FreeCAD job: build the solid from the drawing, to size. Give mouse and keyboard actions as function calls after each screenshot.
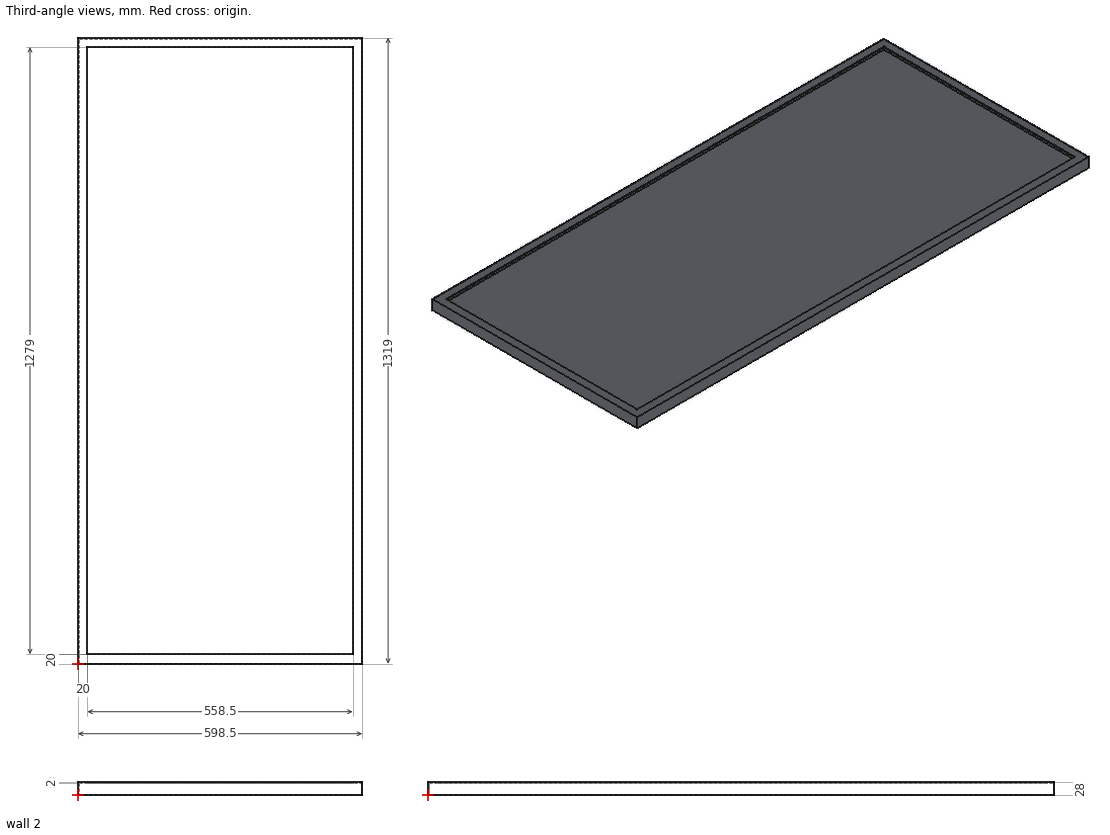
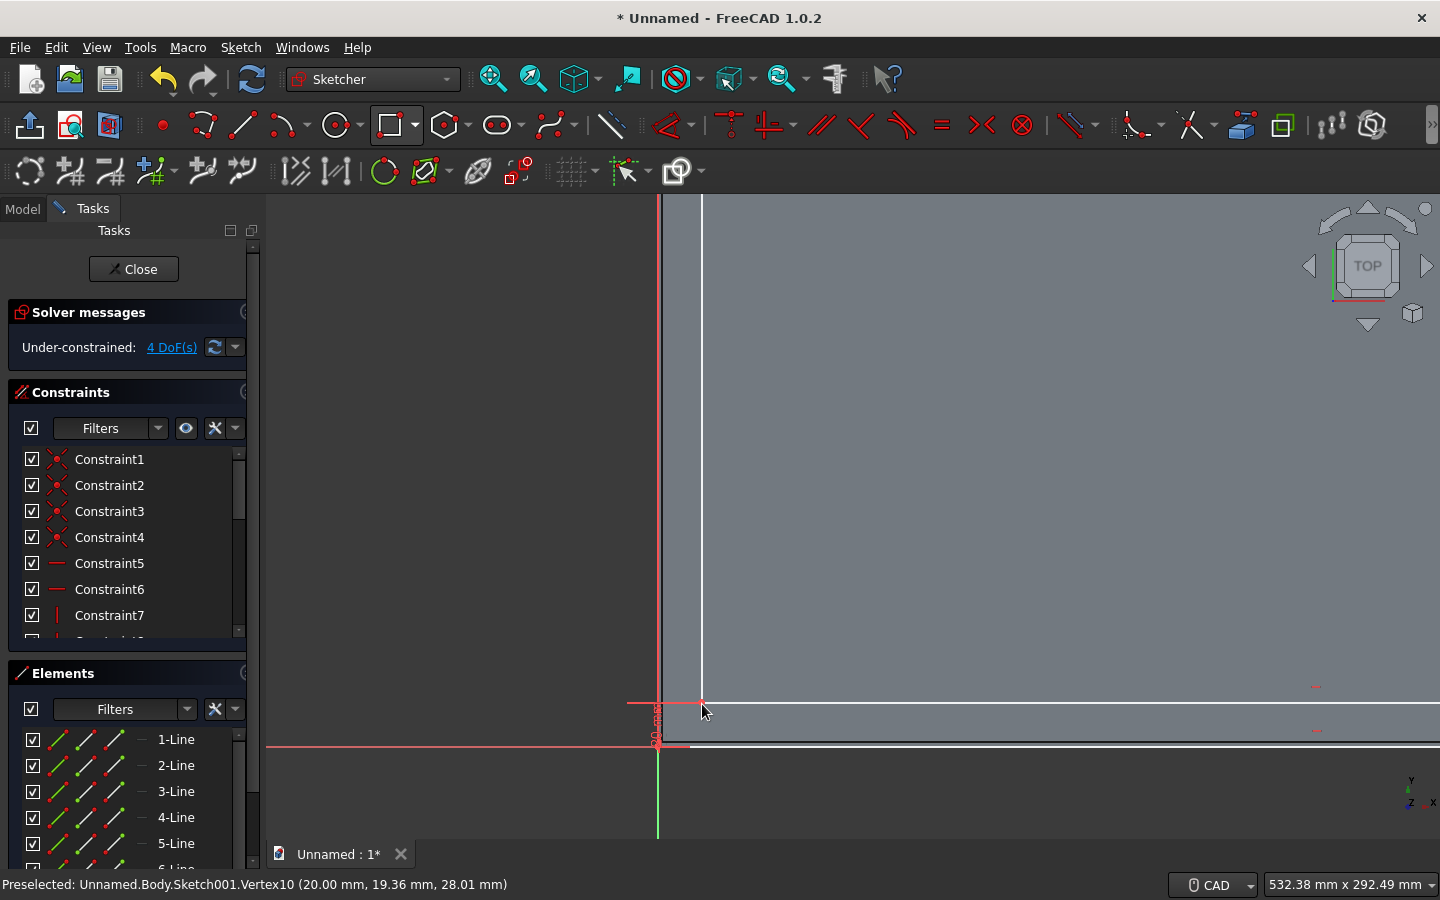
scroll(701, 708, down, 10)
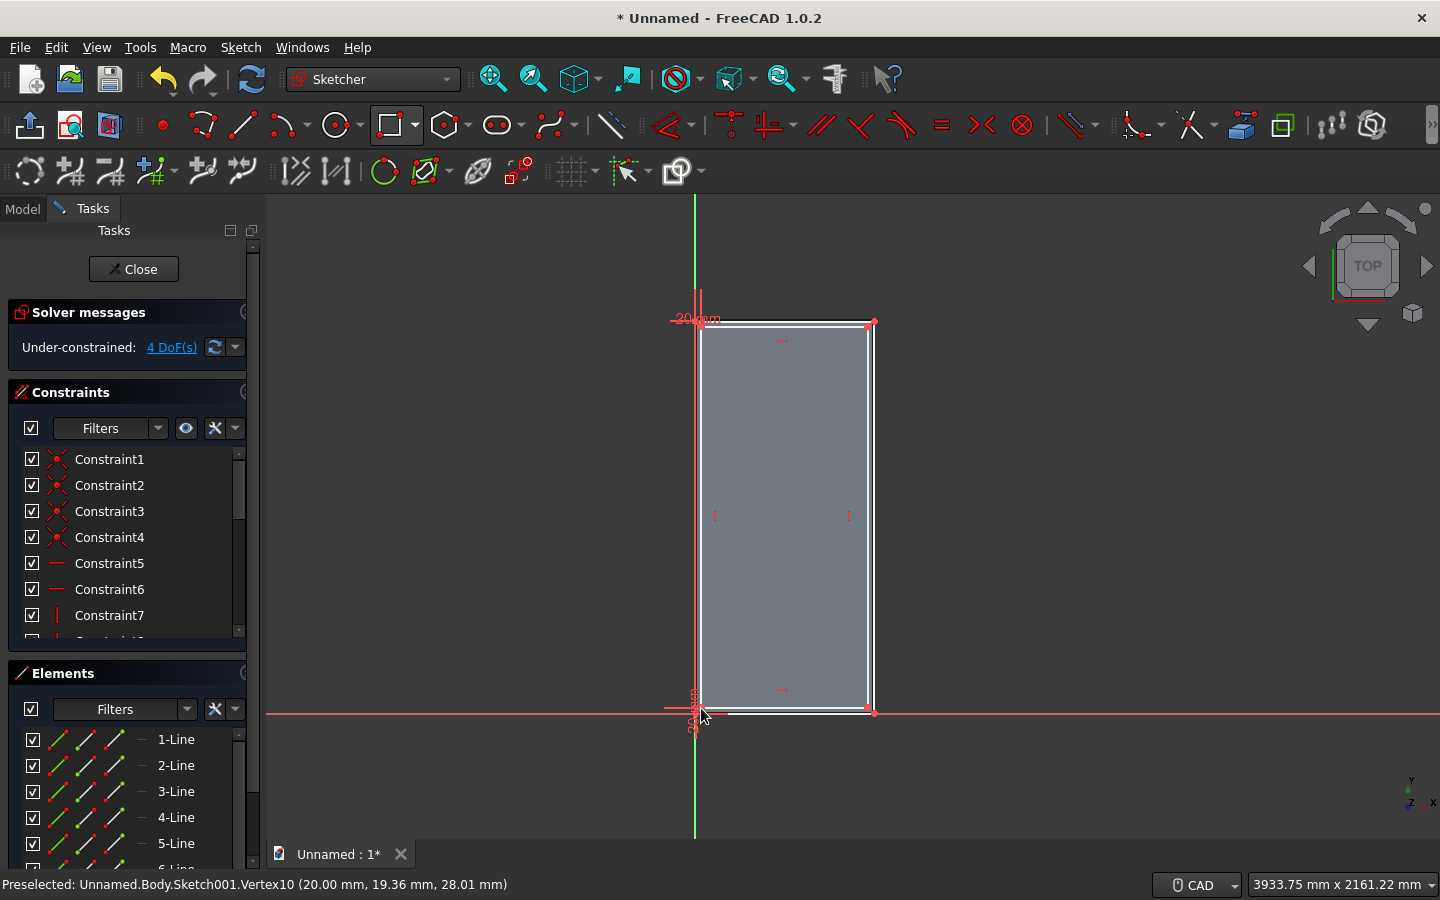
scroll(874, 596, up, 5)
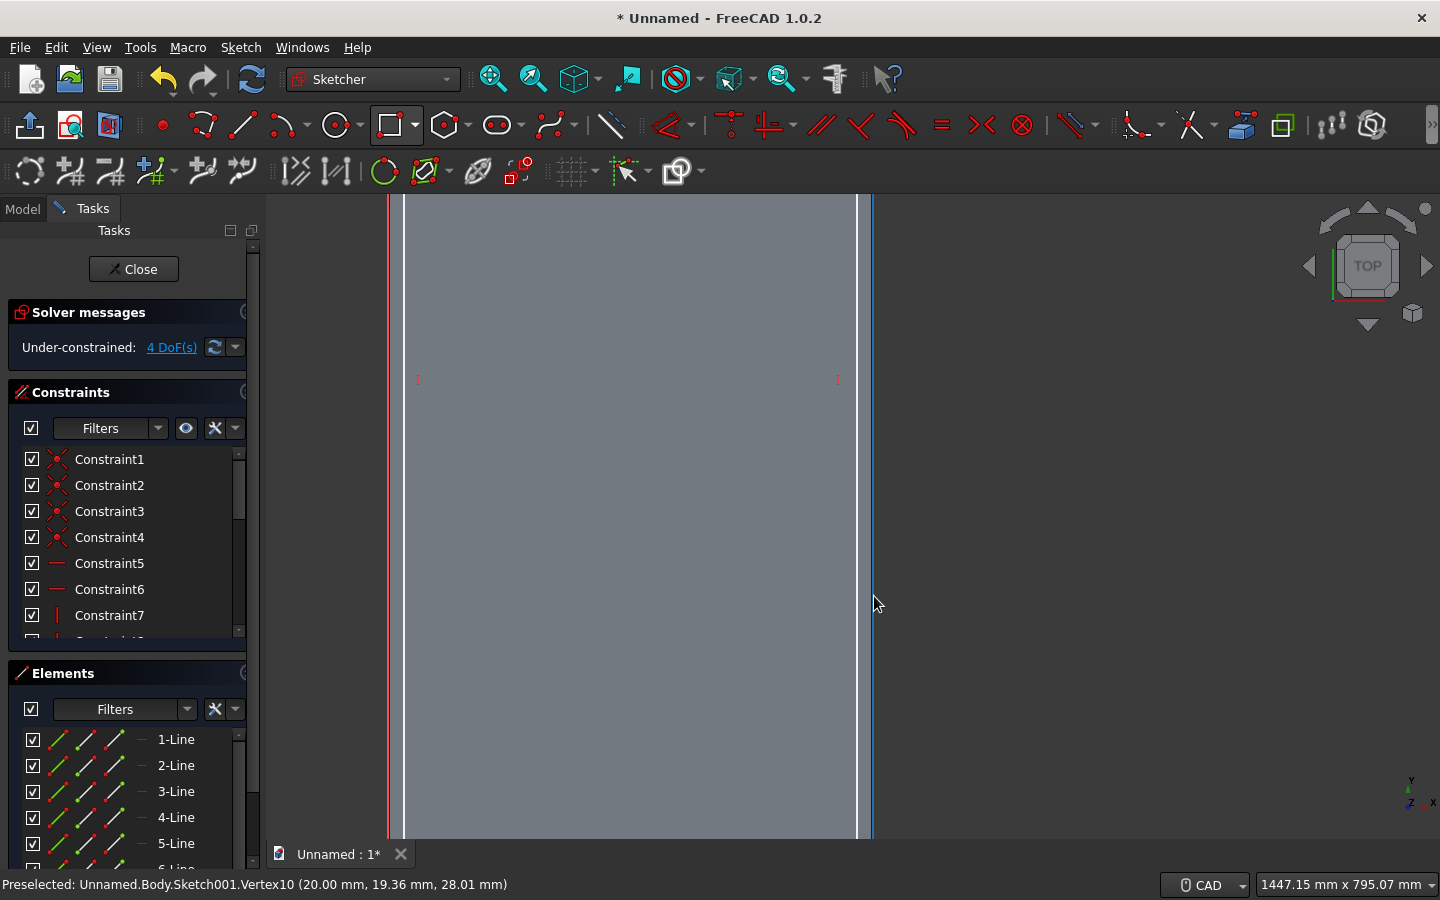
click(873, 596)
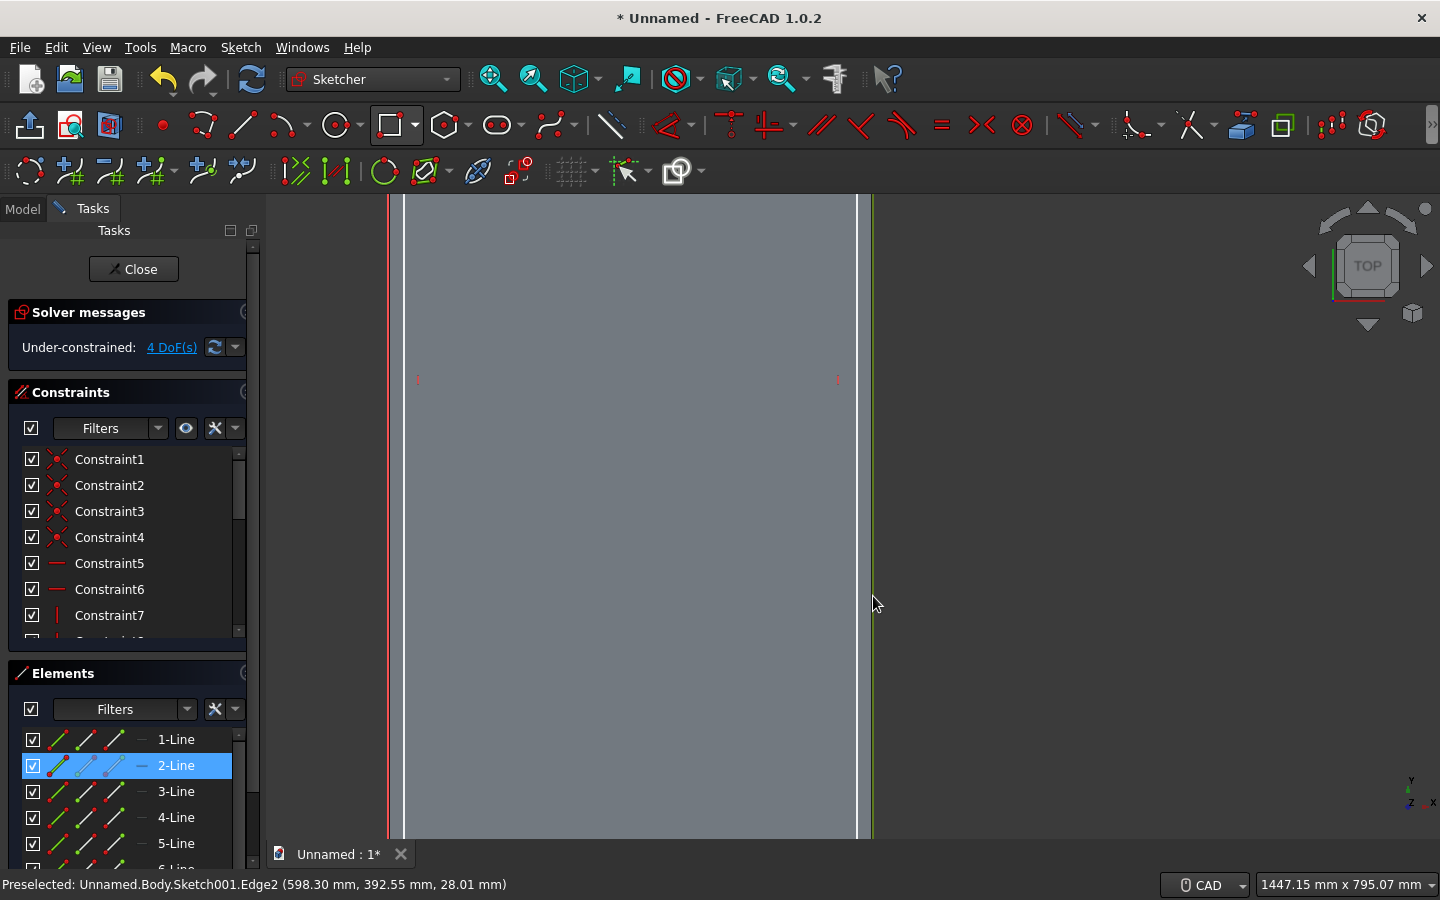
click(694, 126)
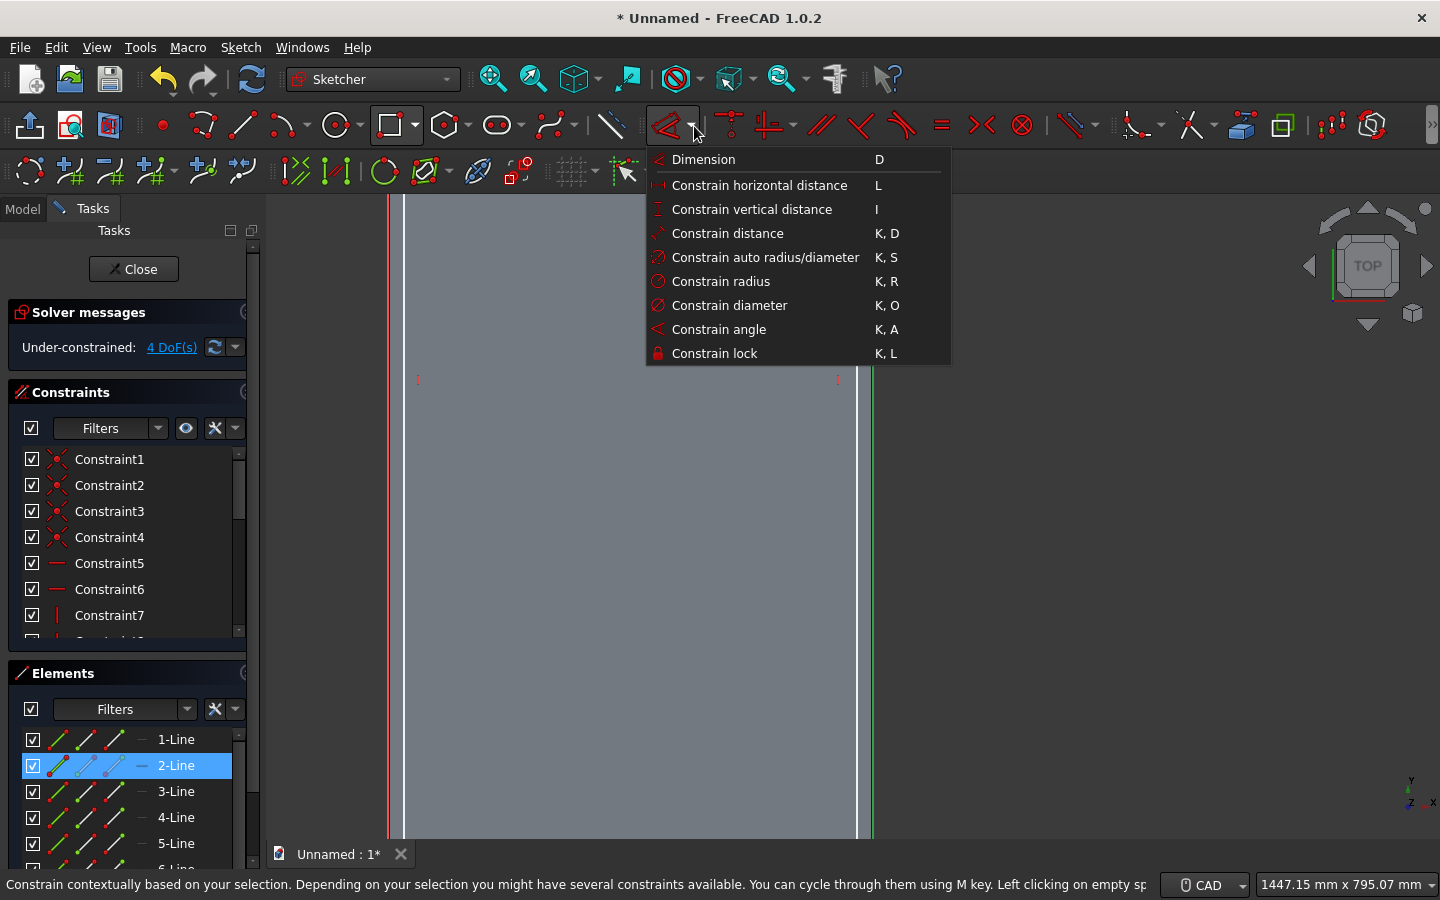
click(799, 209)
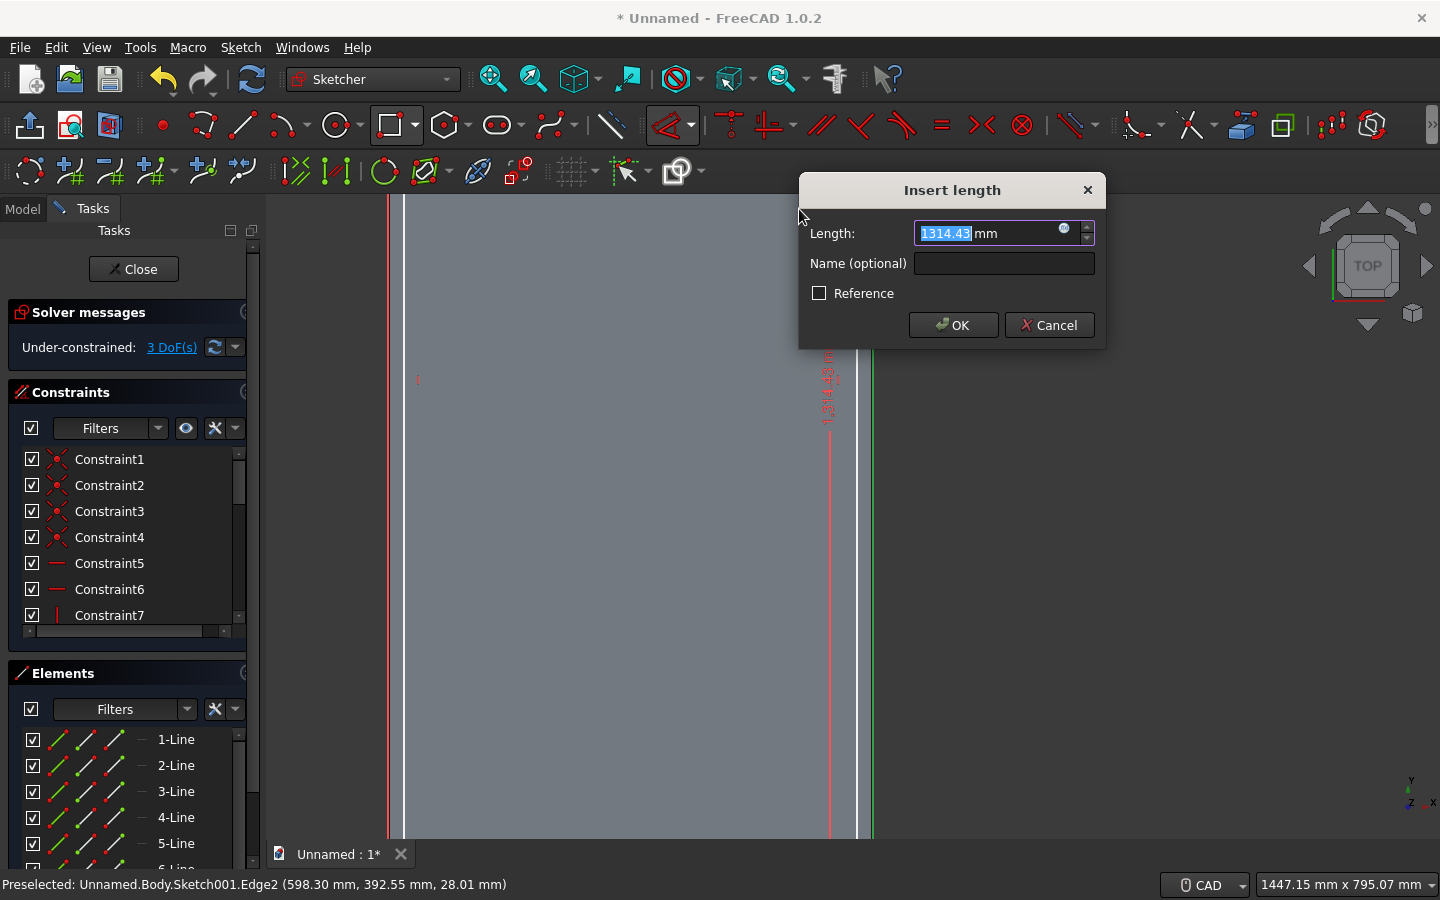
text(1319)
key(Return)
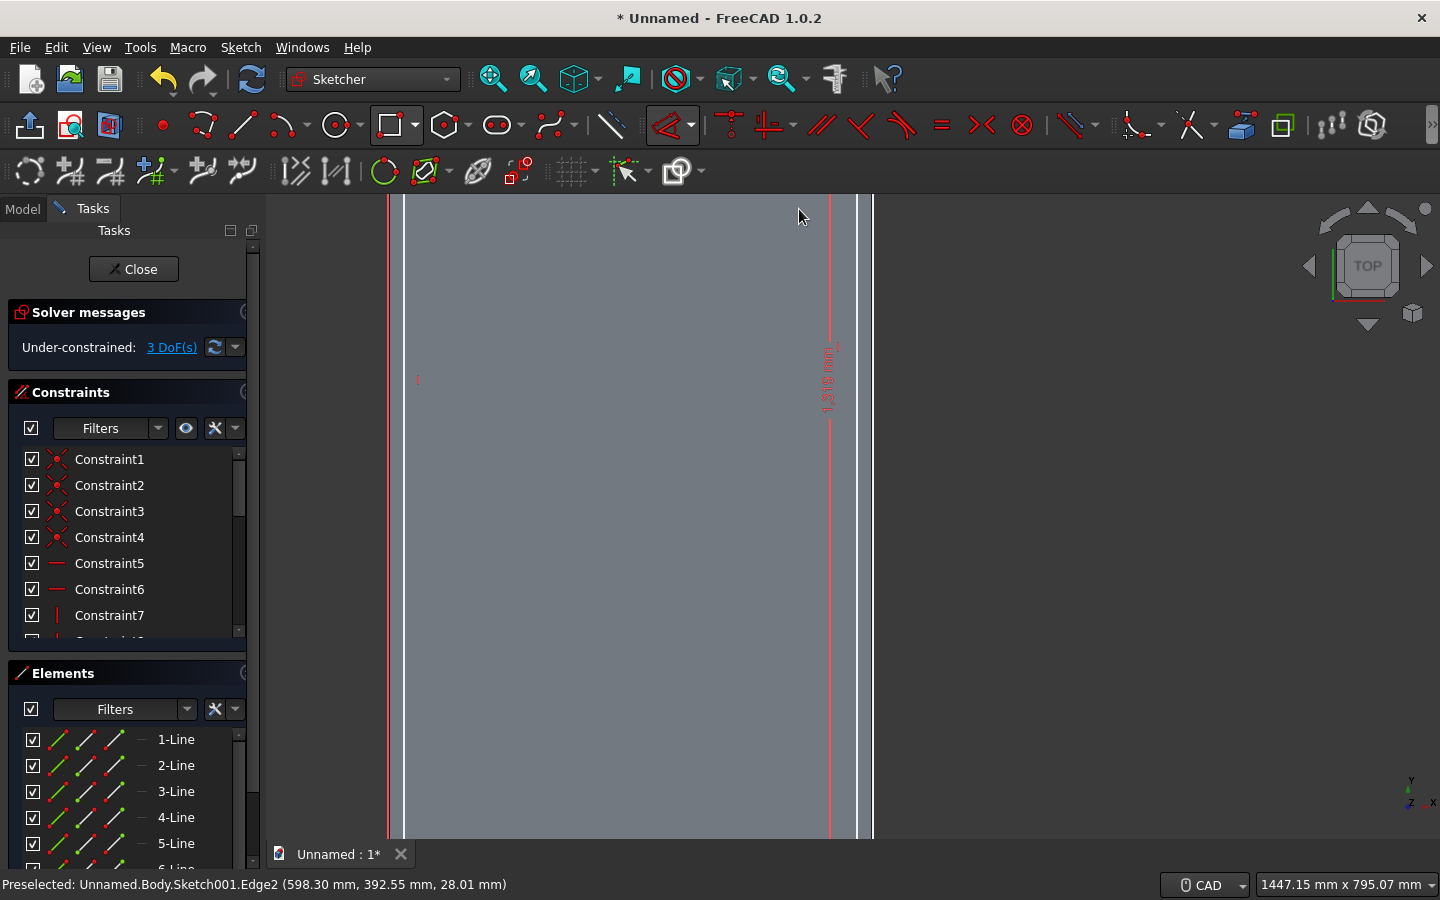
click(404, 588)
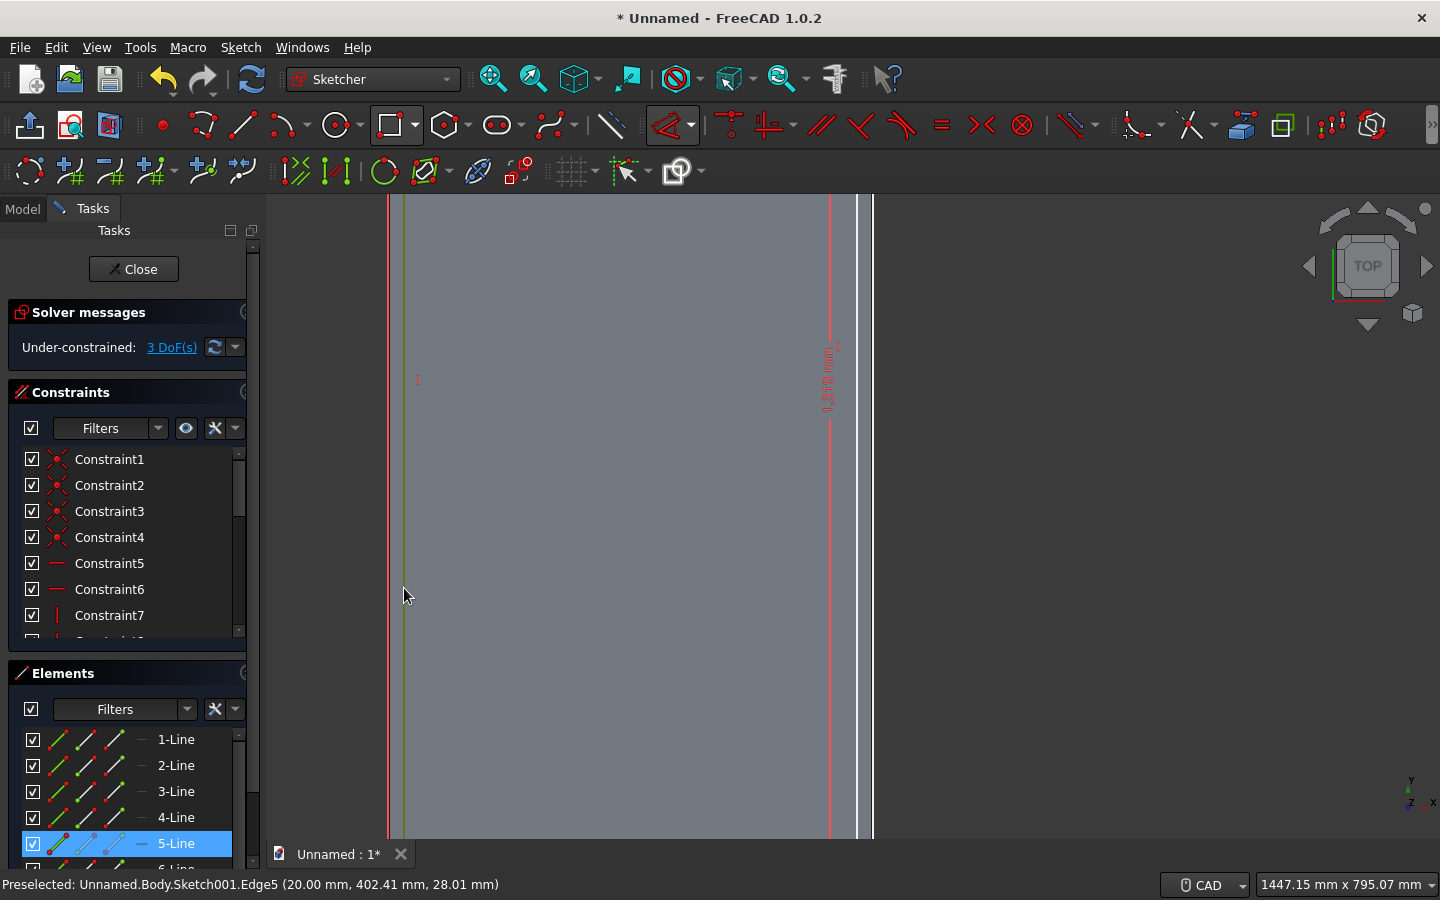
key(i)